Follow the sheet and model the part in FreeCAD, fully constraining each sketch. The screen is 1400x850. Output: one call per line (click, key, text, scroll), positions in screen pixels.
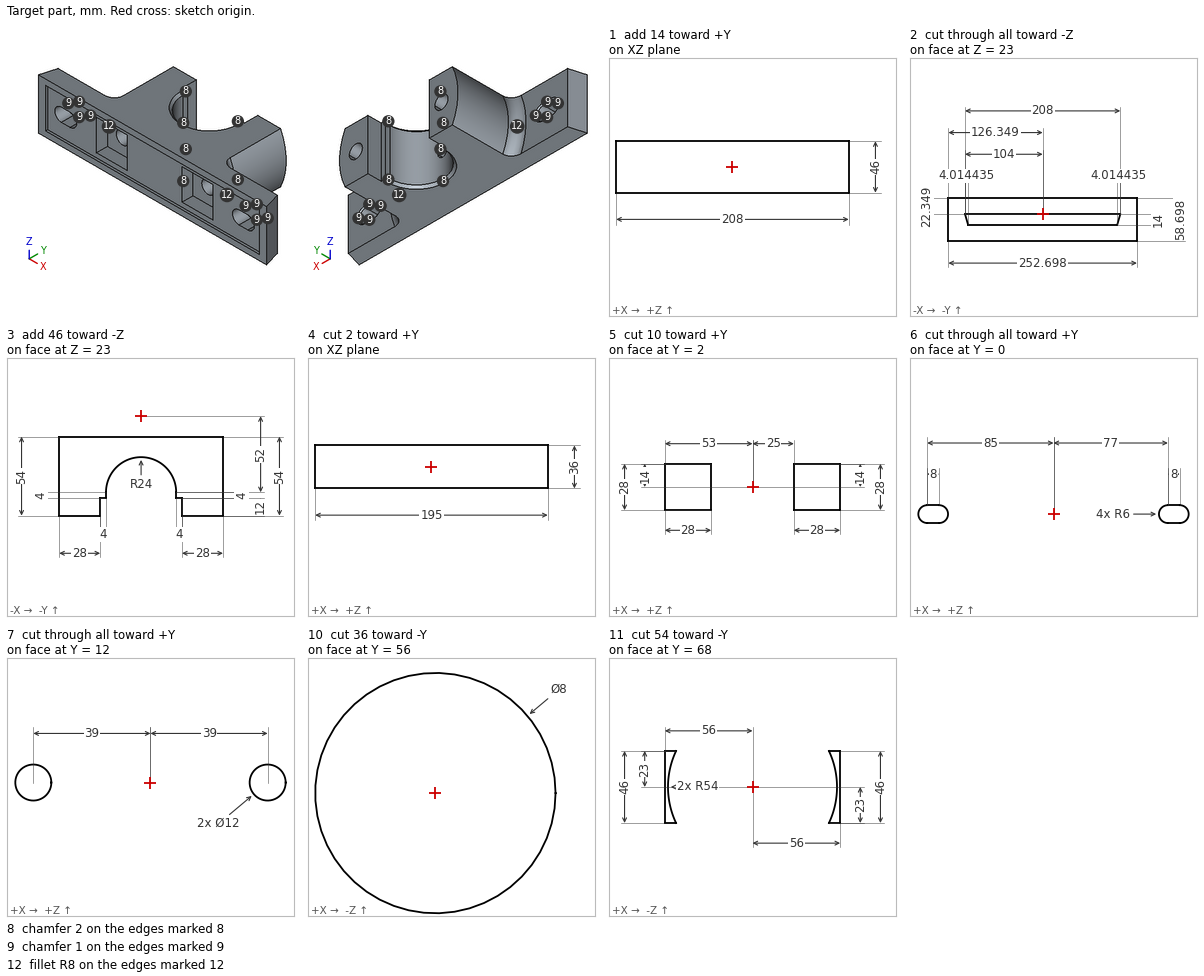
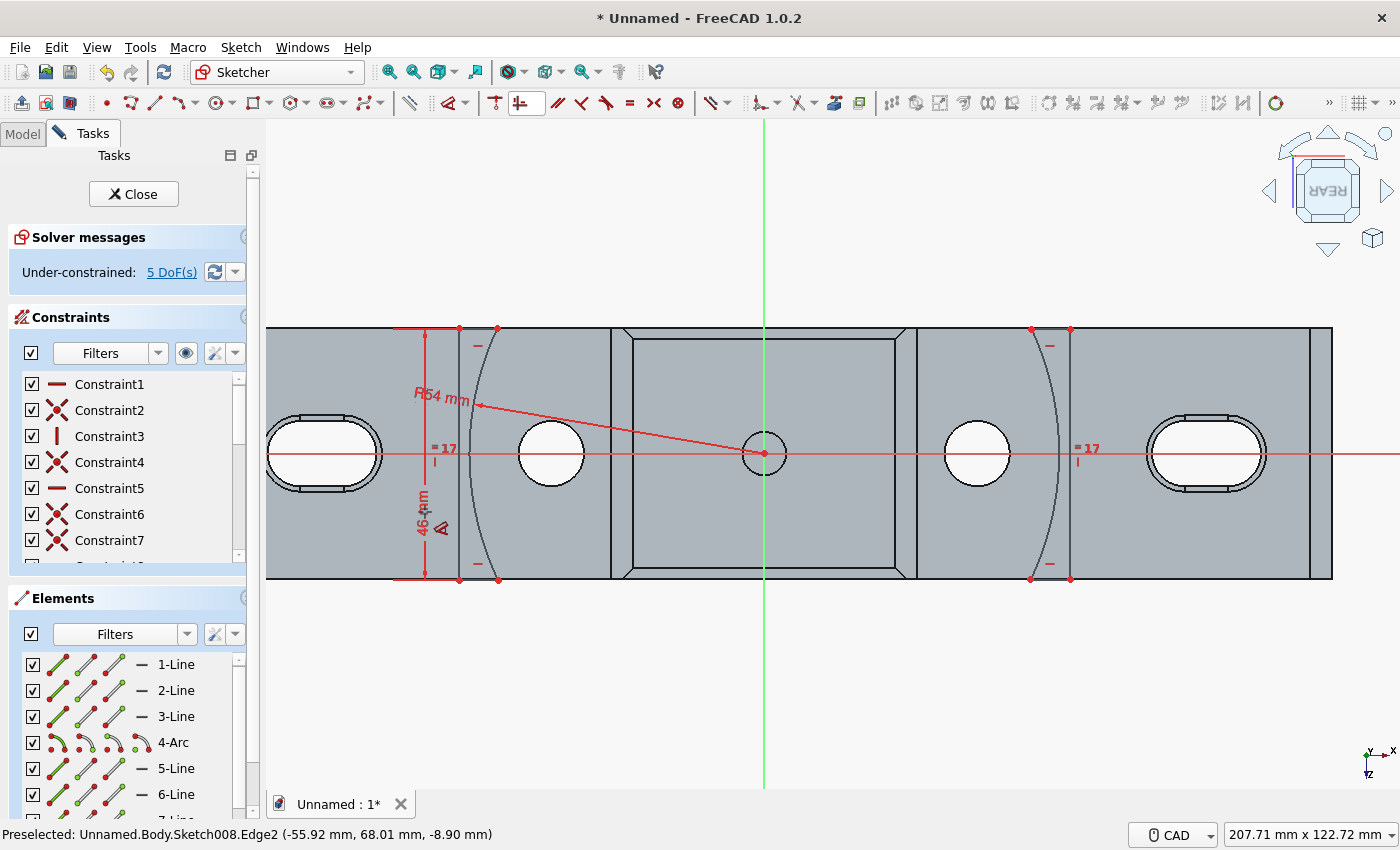
click(1070, 505)
click(1104, 397)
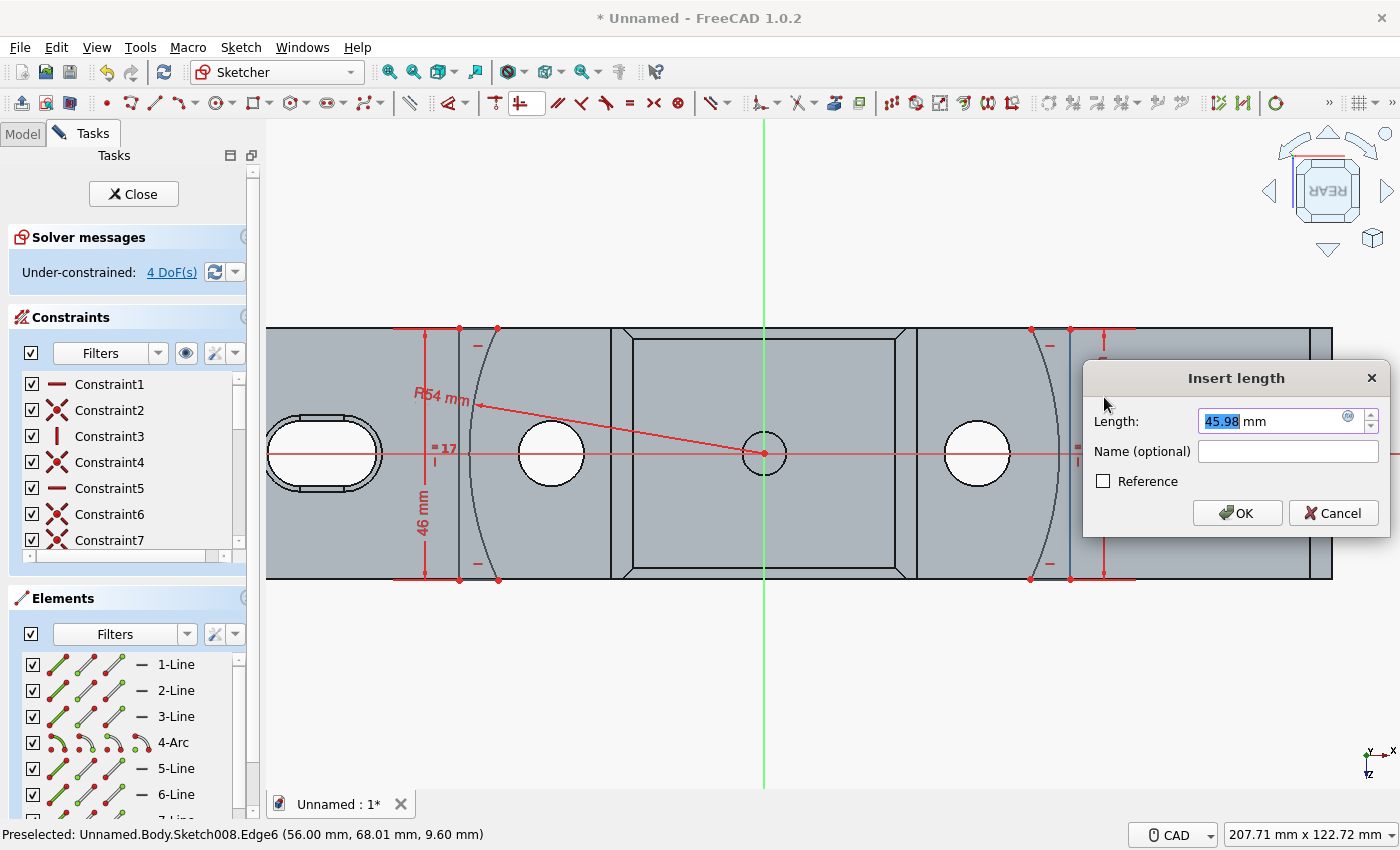
text(46)
key(Return)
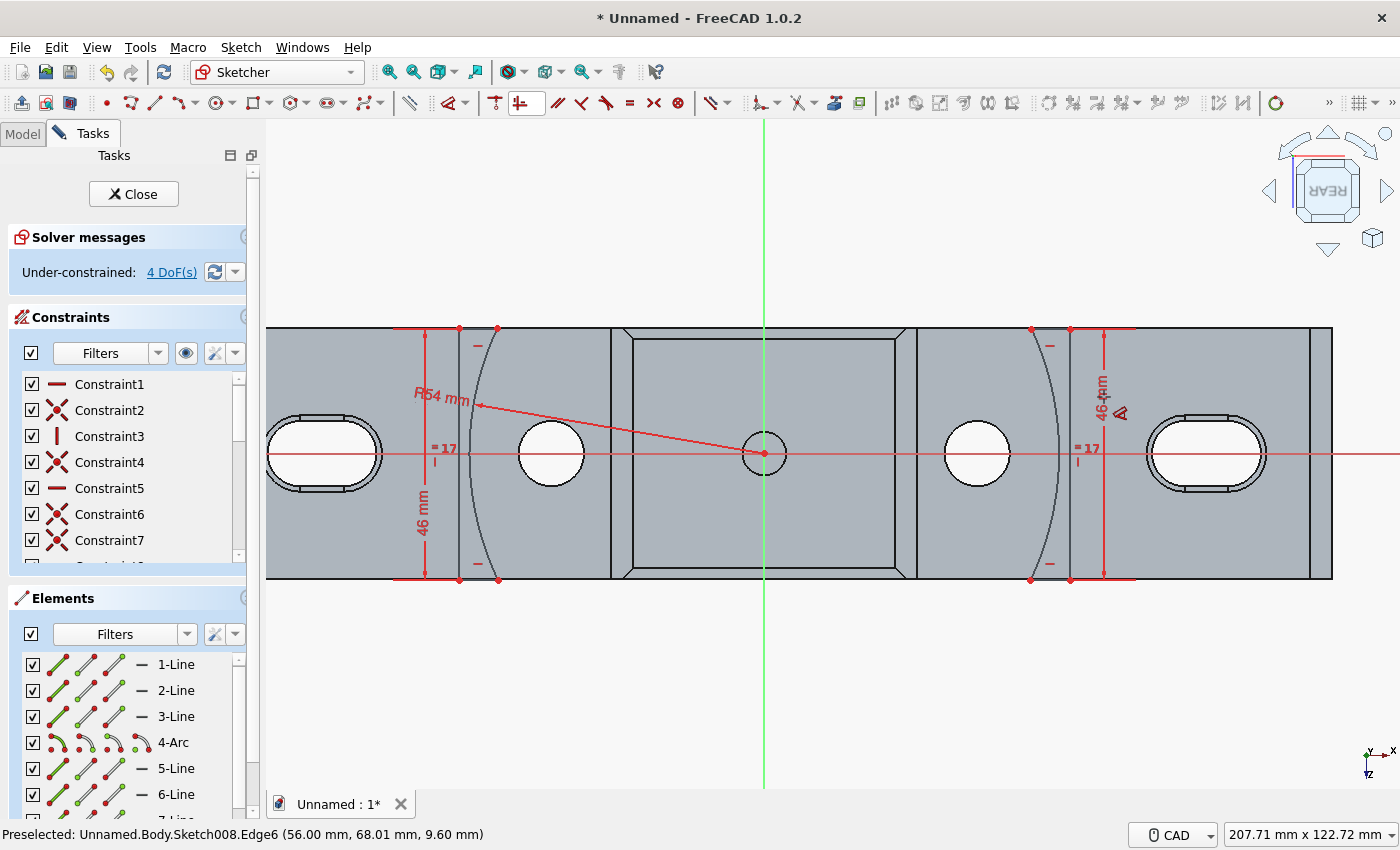
click(497, 329)
click(798, 391)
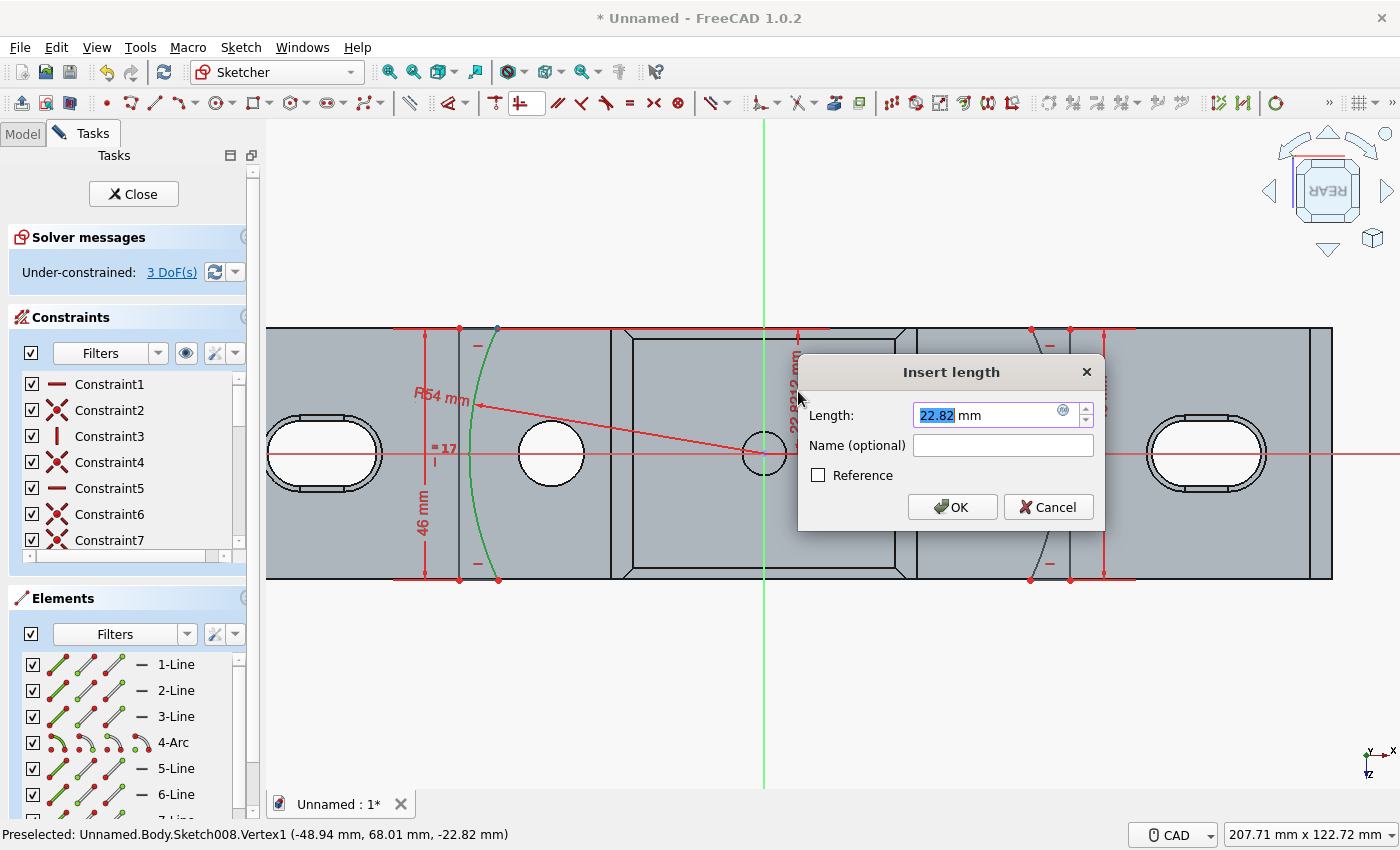
text(23)
key(Return)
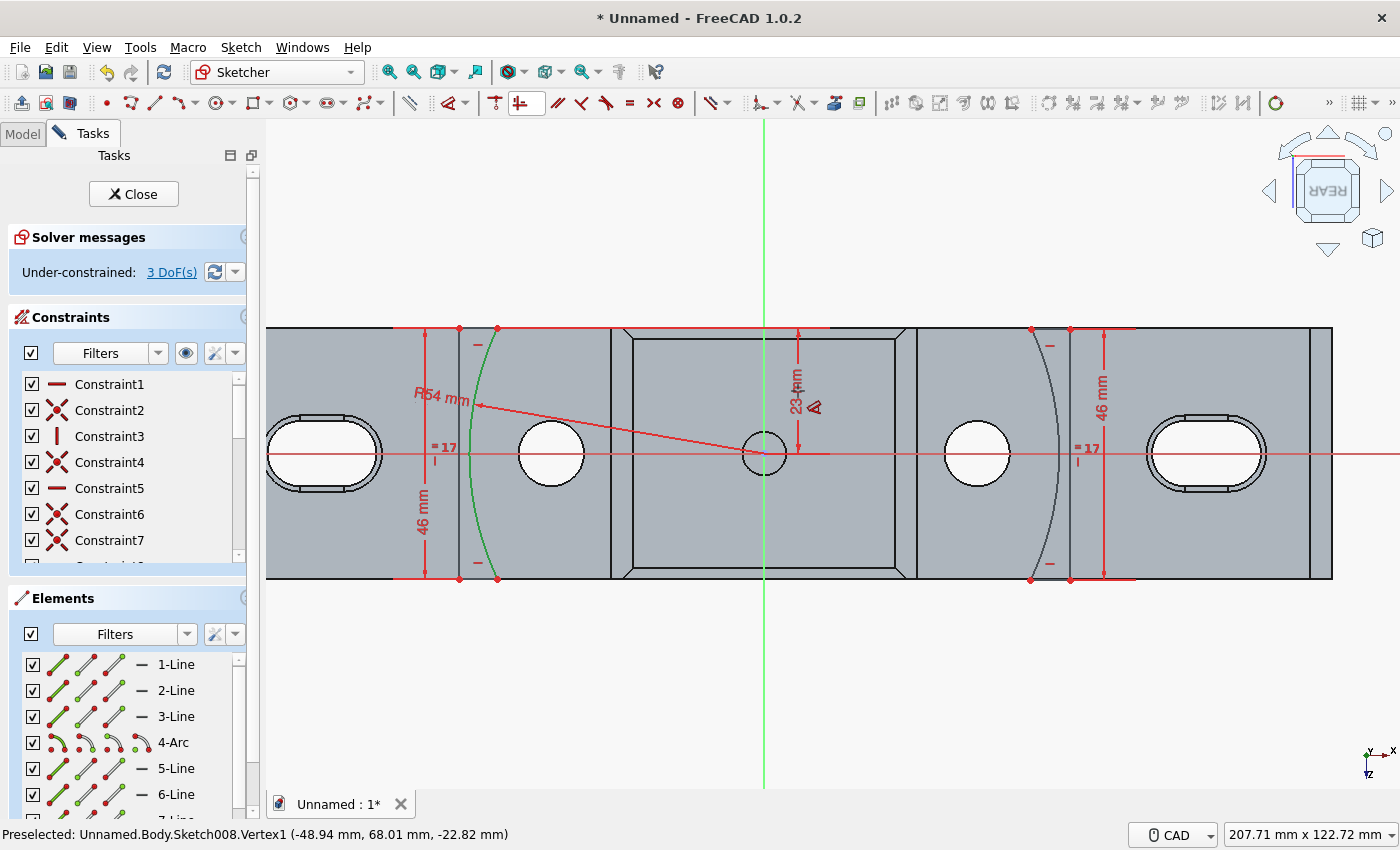
click(459, 328)
click(612, 294)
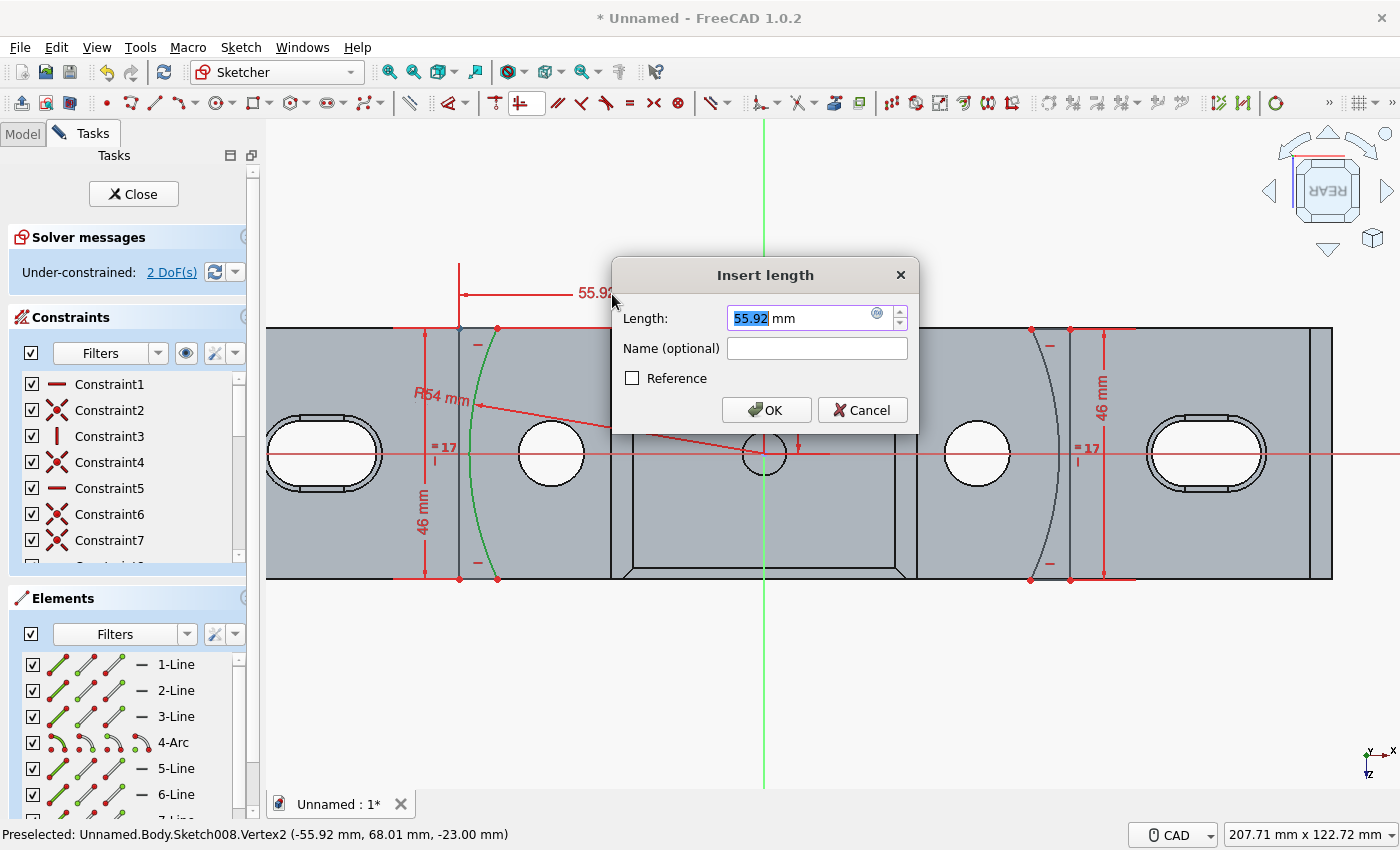
text(56)
key(Return)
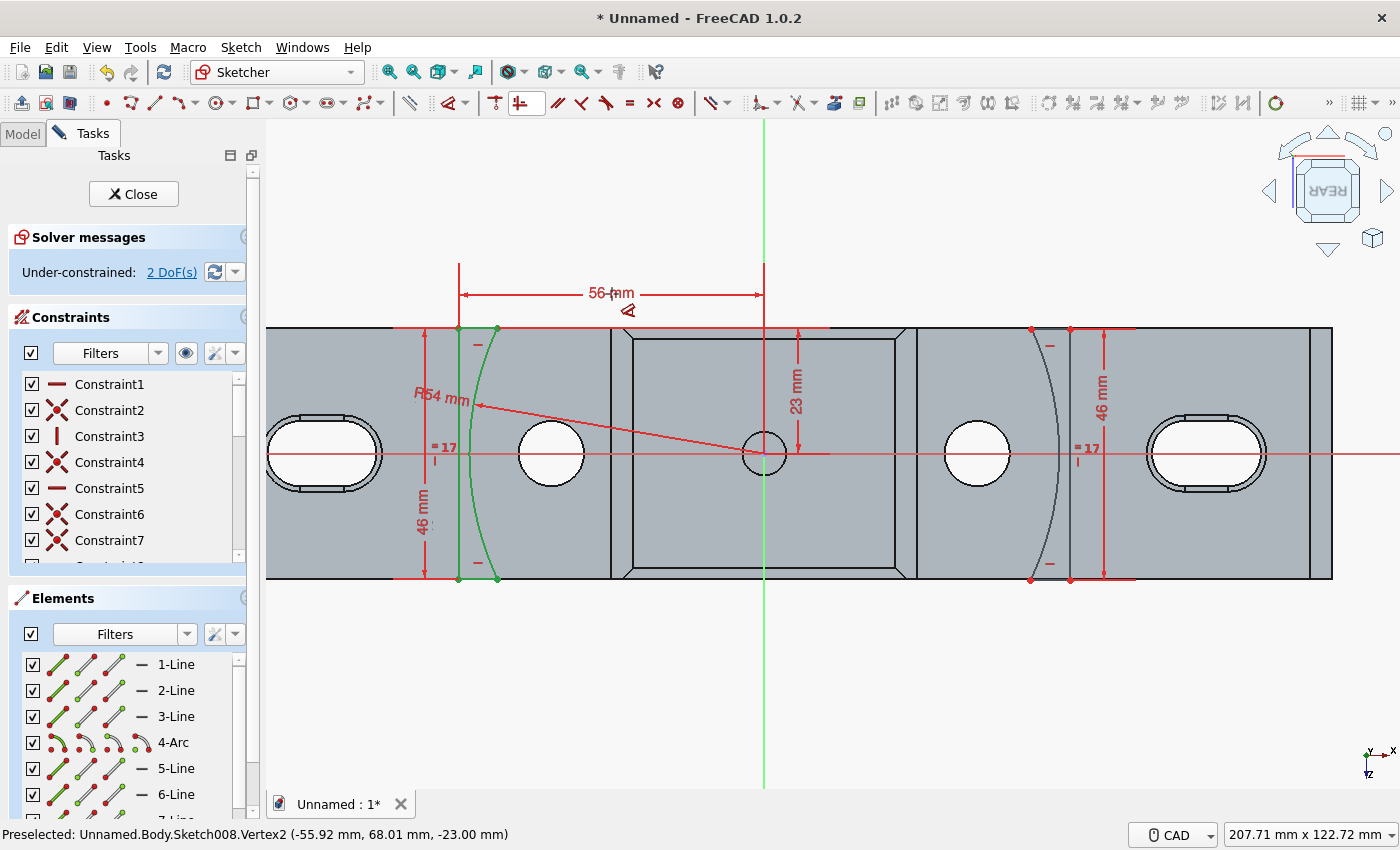
click(1031, 580)
click(730, 517)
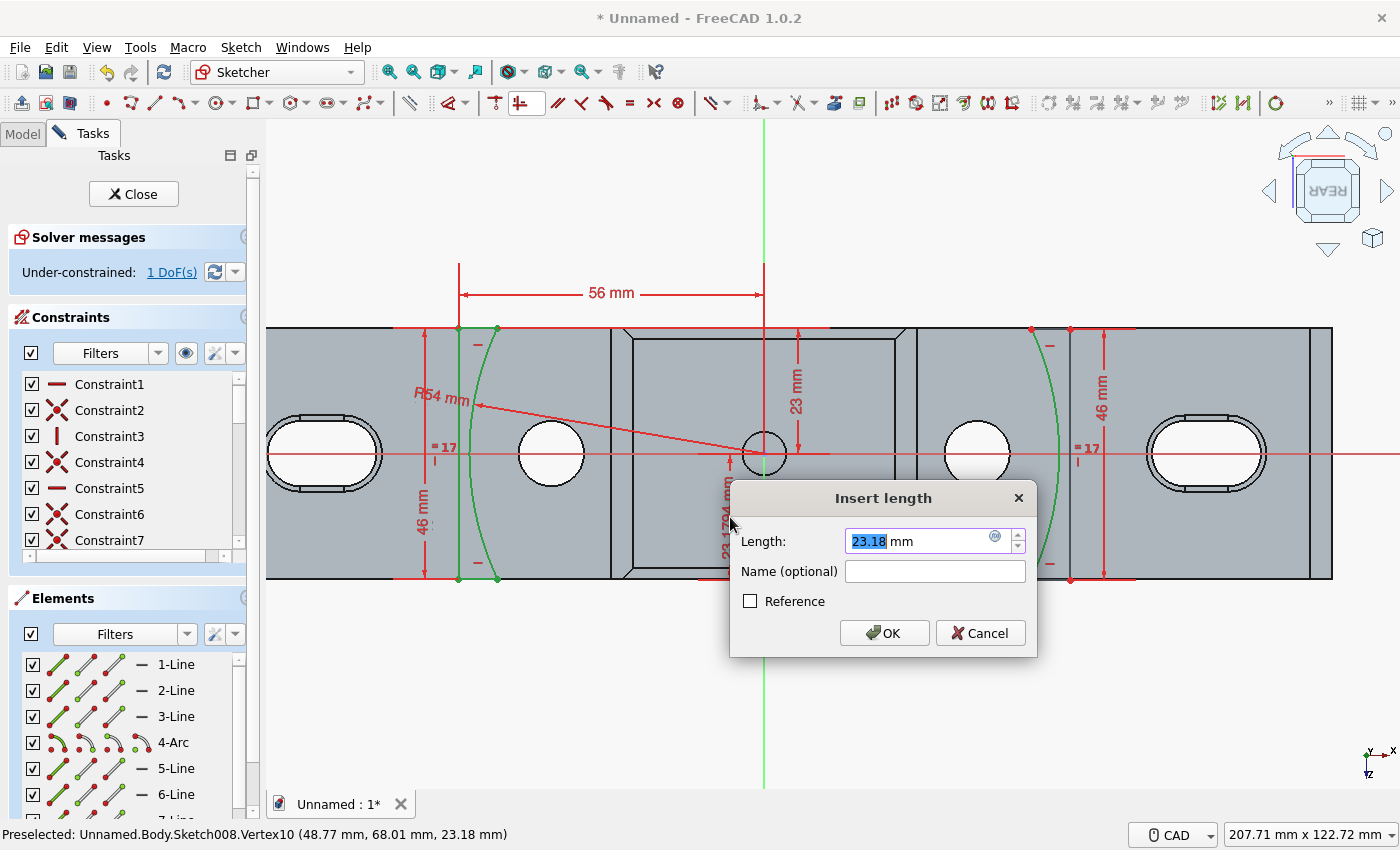
text(23)
key(Return)